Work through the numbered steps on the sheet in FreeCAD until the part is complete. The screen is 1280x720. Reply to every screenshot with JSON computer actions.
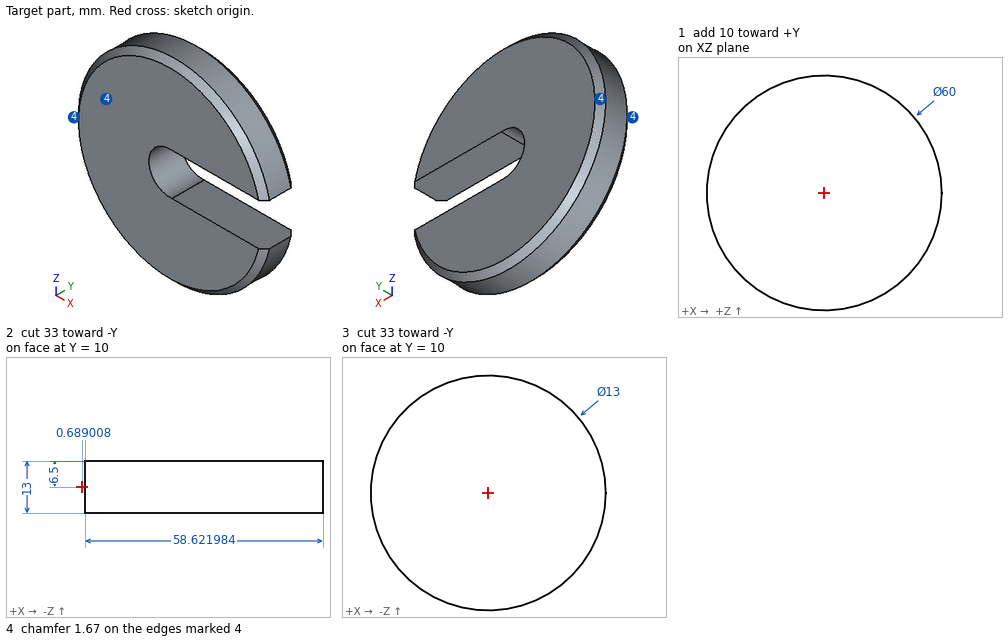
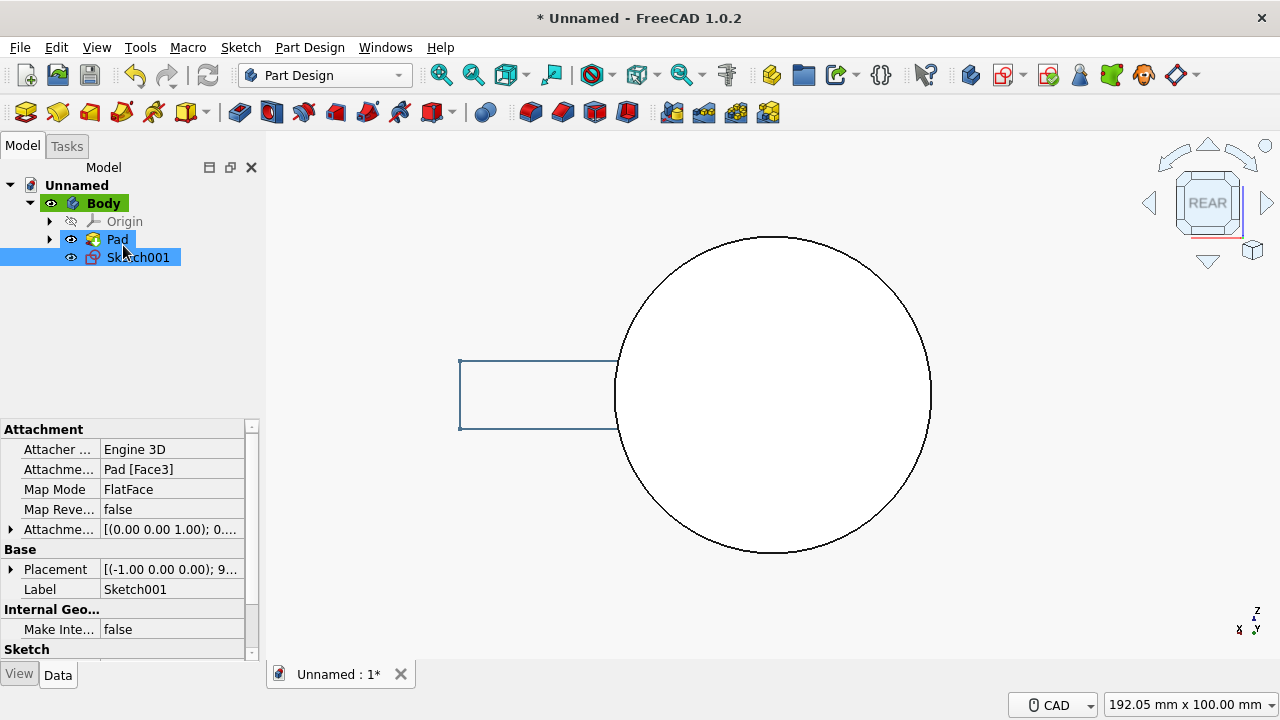
{"action": "left_click", "coordinate": [240, 112]}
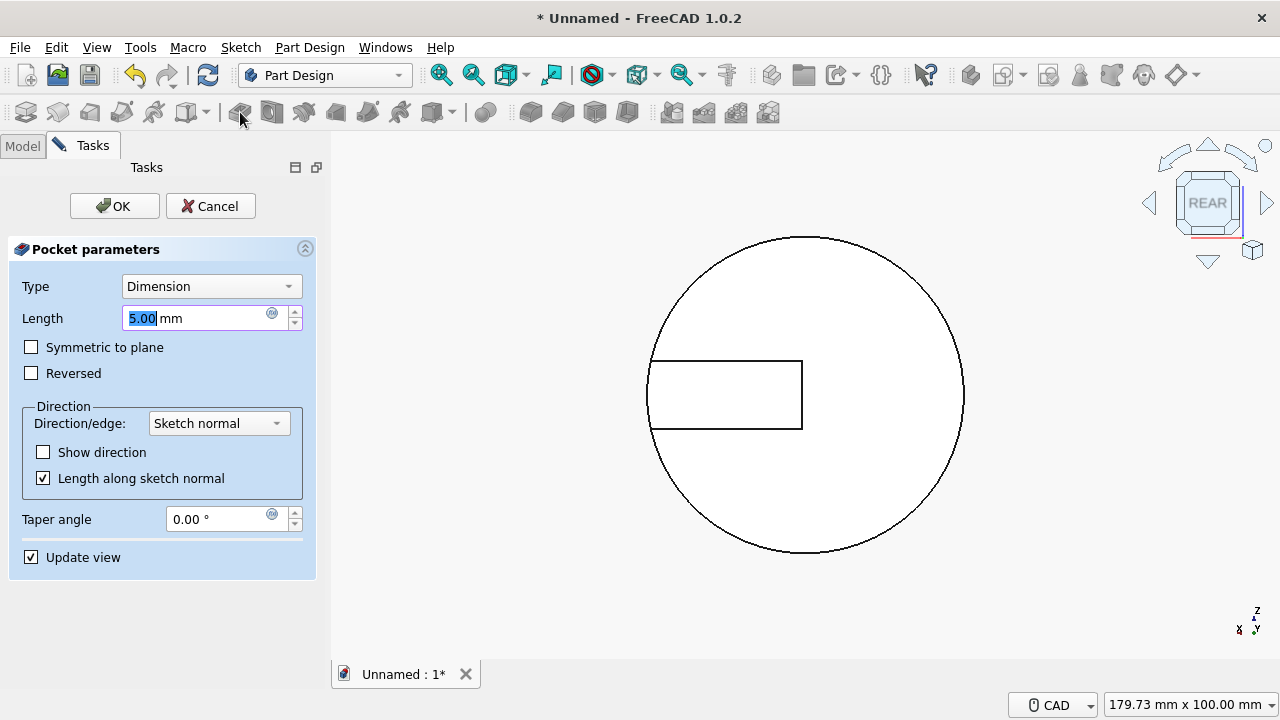
{"action": "type", "text": "33"}
{"action": "key", "text": "Tab"}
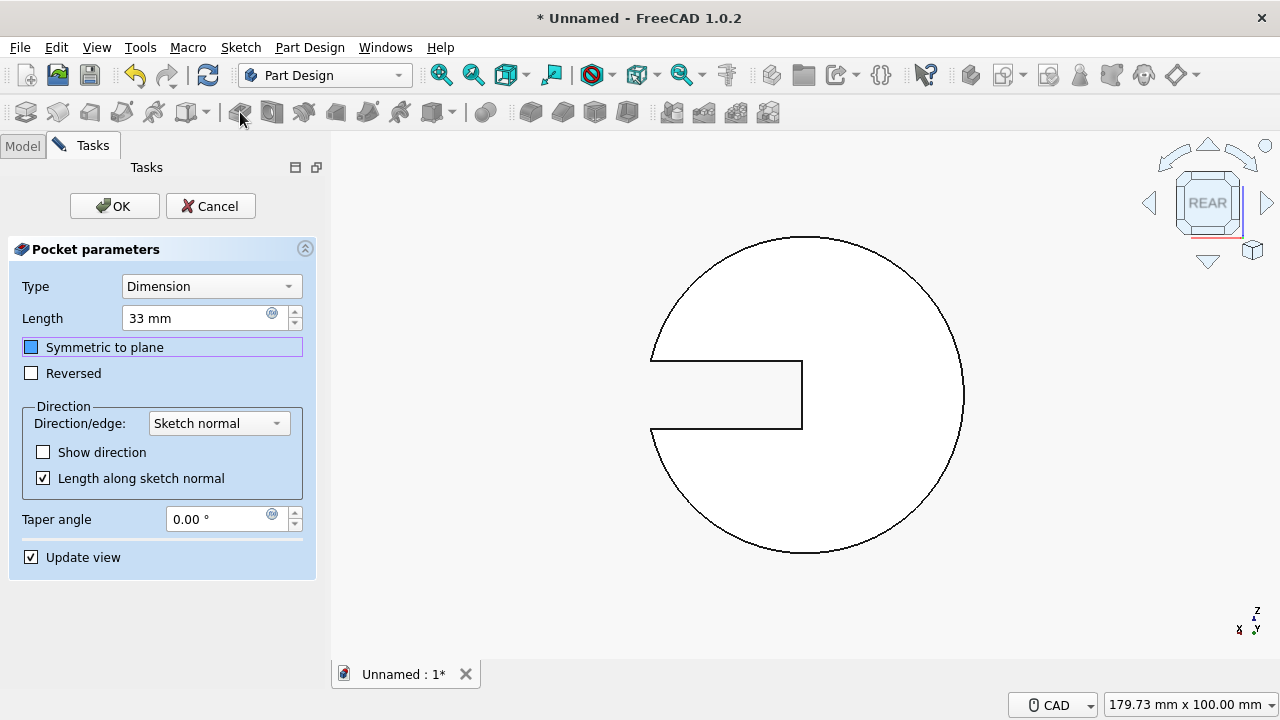
{"action": "left_click", "coordinate": [115, 206]}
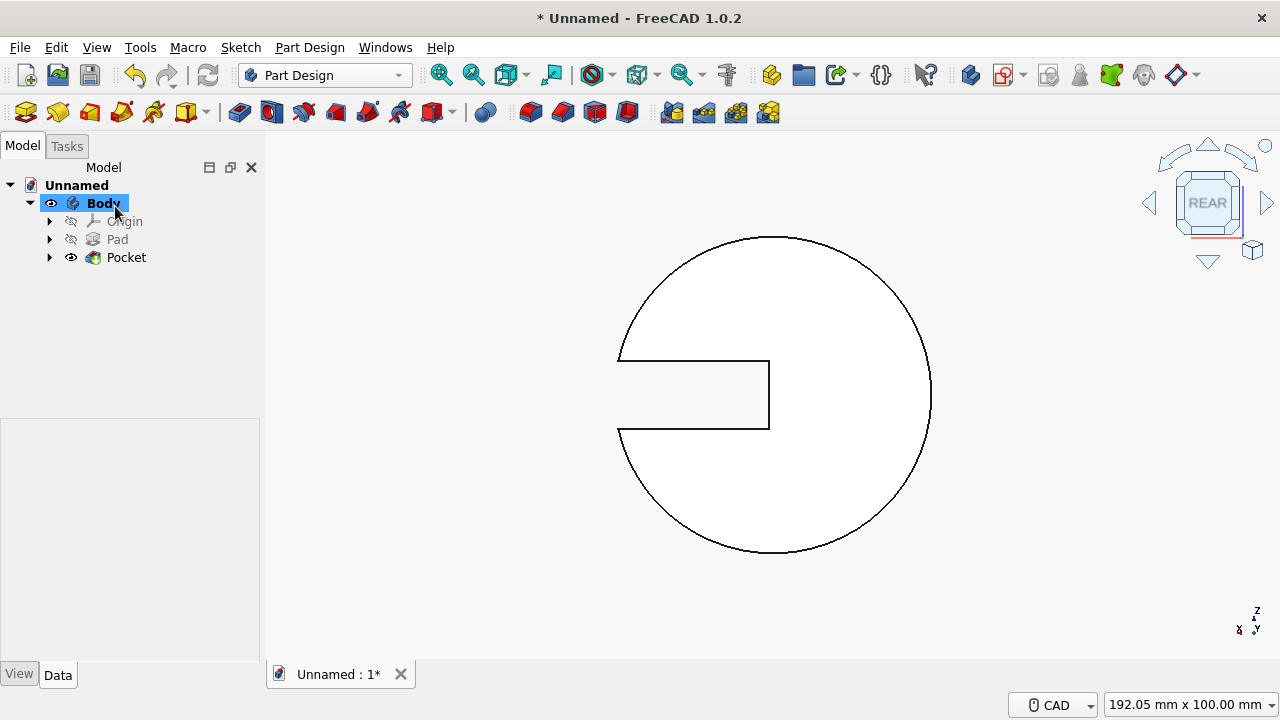
{"action": "left_click", "coordinate": [864, 394]}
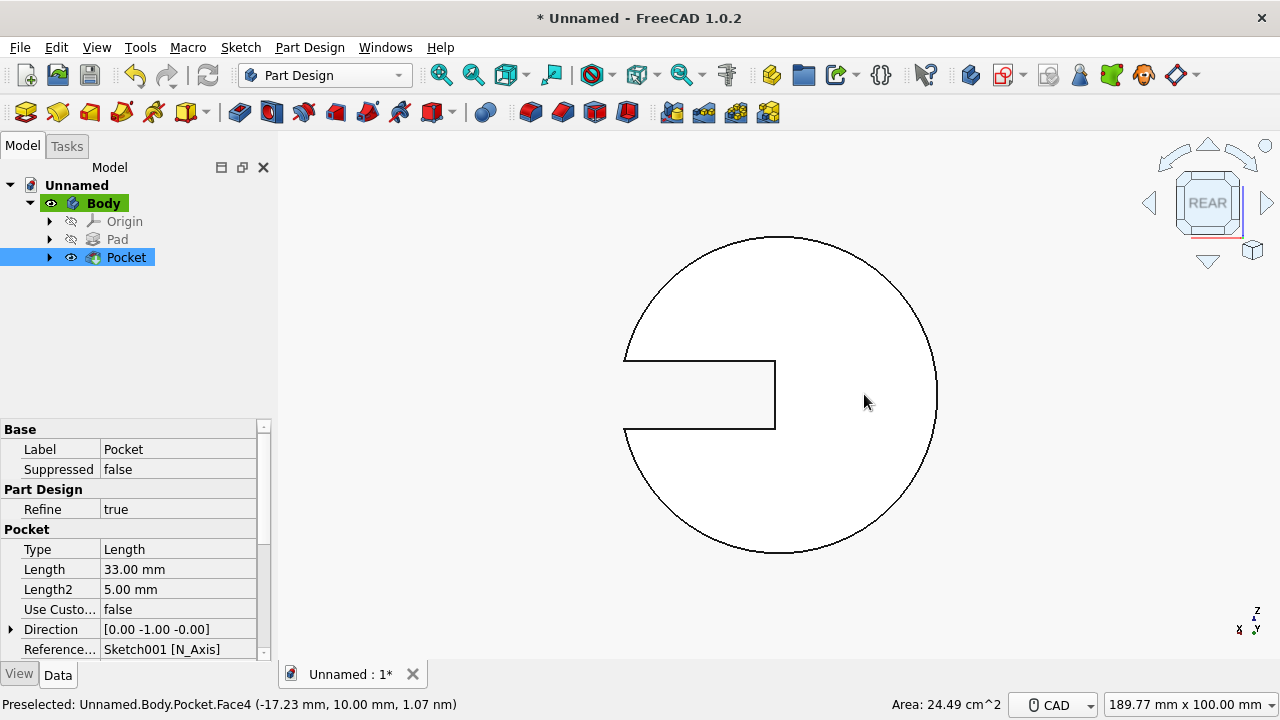
{"action": "left_click", "coordinate": [1004, 76]}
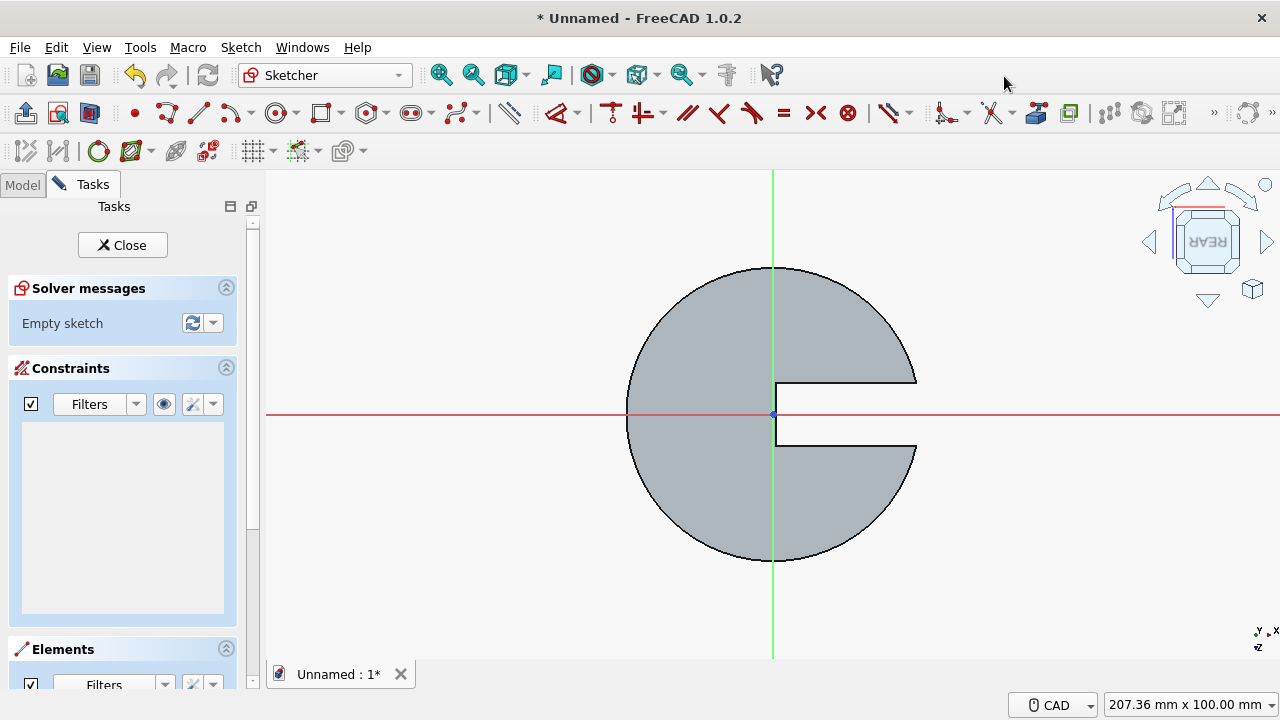
{"action": "scroll", "coordinate": [790, 414], "scroll_direction": "up", "scroll_amount": 8}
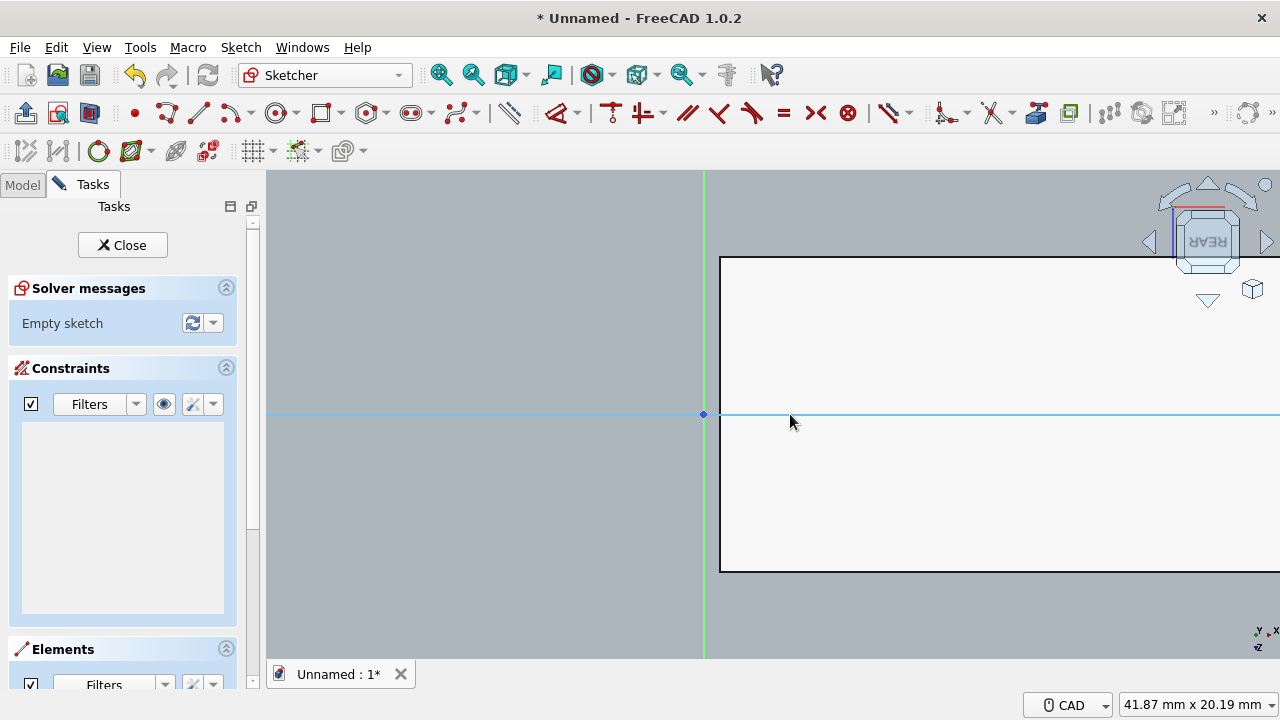
{"action": "left_click", "coordinate": [276, 114]}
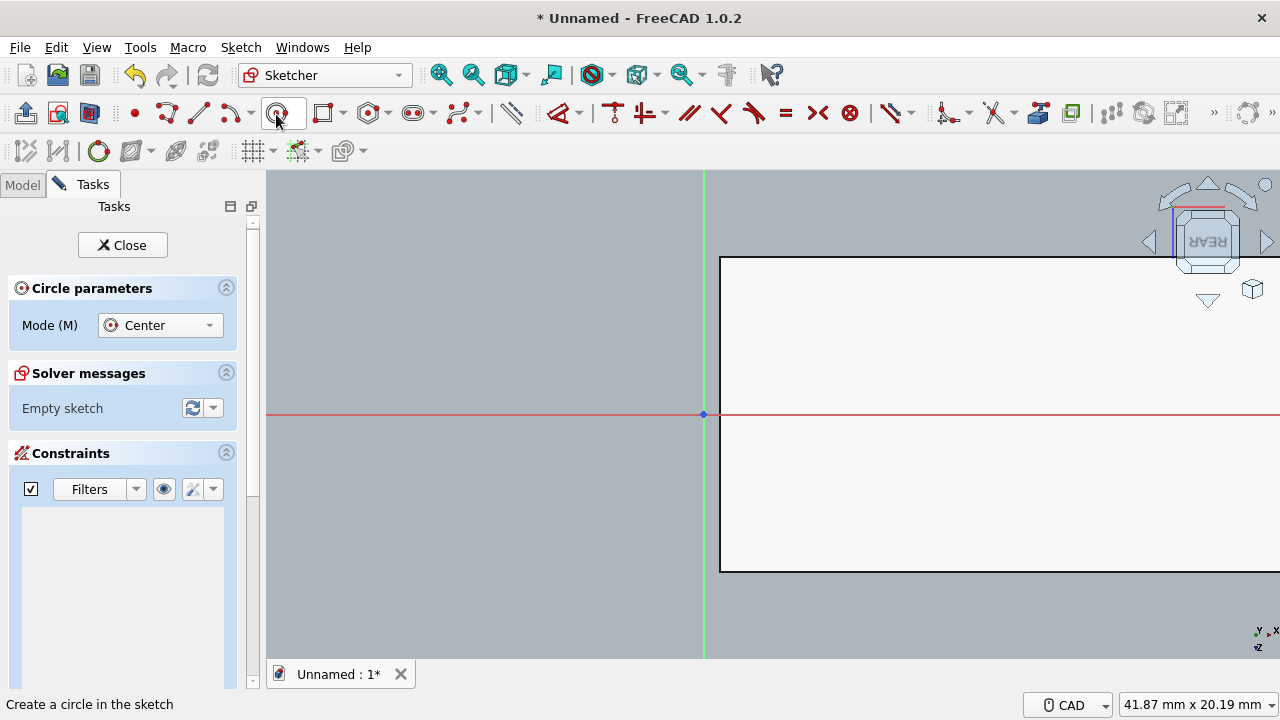
{"action": "left_click", "coordinate": [704, 414]}
{"action": "mouse_move", "coordinate": [815, 303]}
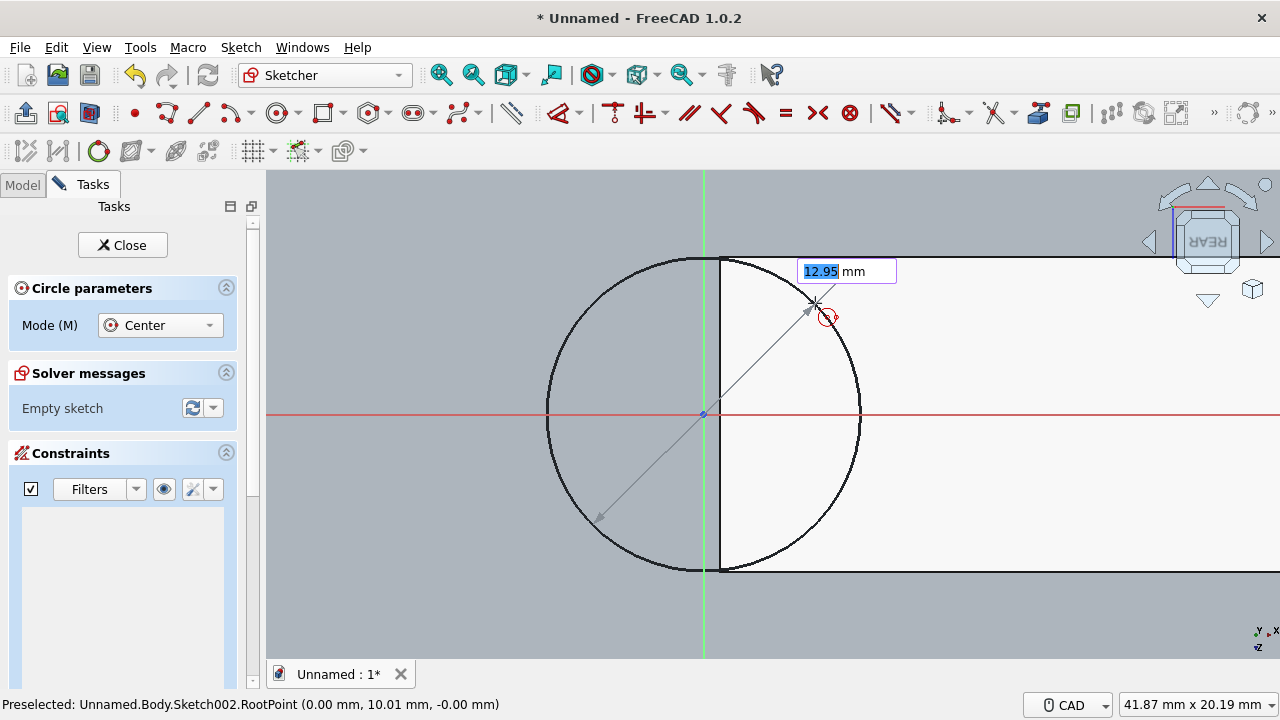
{"action": "type", "text": "13"}
{"action": "key", "text": "Return"}
{"action": "key", "text": "Escape"}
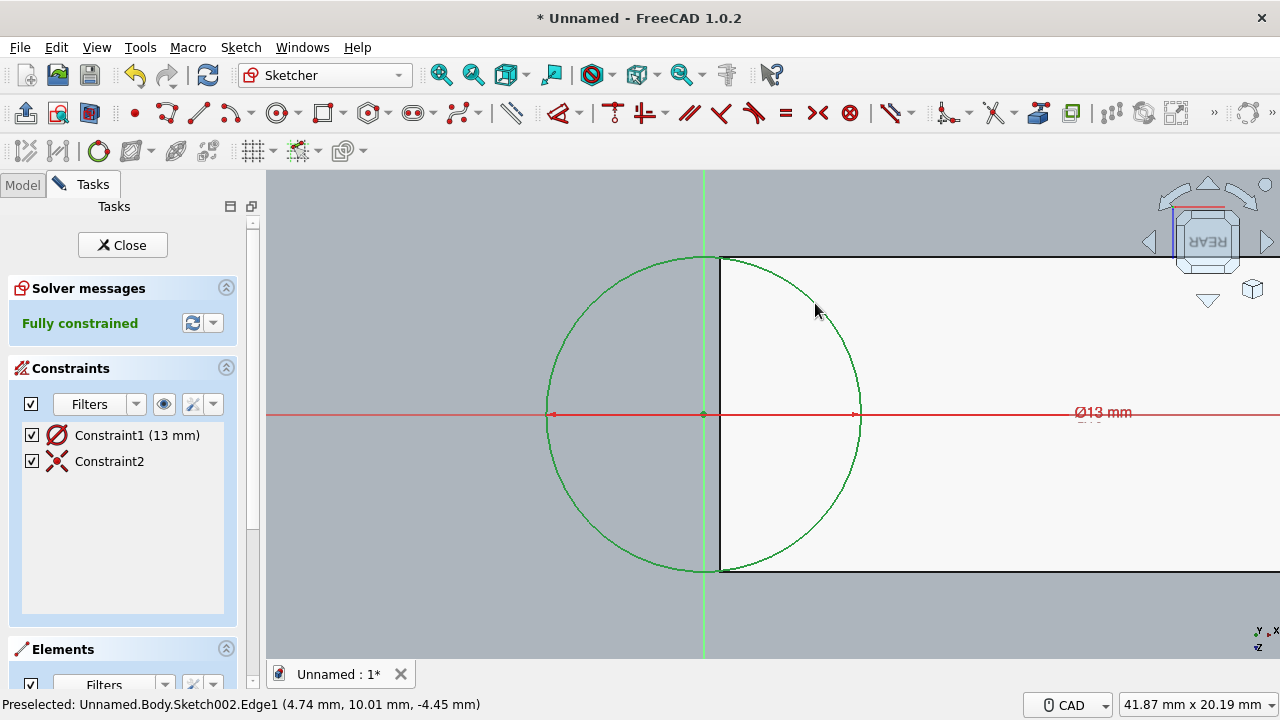
{"action": "left_click", "coordinate": [123, 245]}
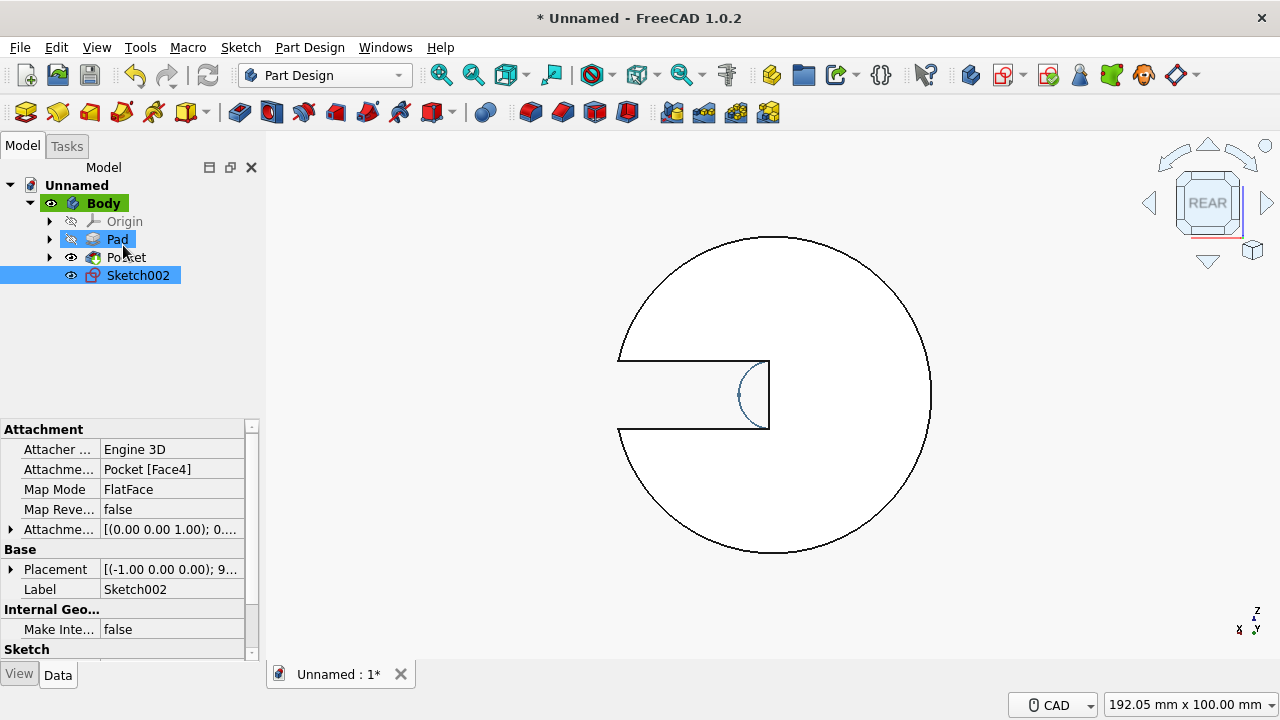
{"action": "left_click", "coordinate": [240, 112]}